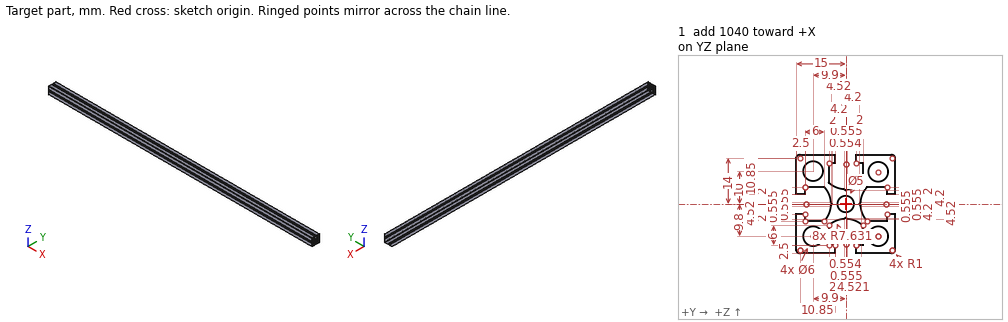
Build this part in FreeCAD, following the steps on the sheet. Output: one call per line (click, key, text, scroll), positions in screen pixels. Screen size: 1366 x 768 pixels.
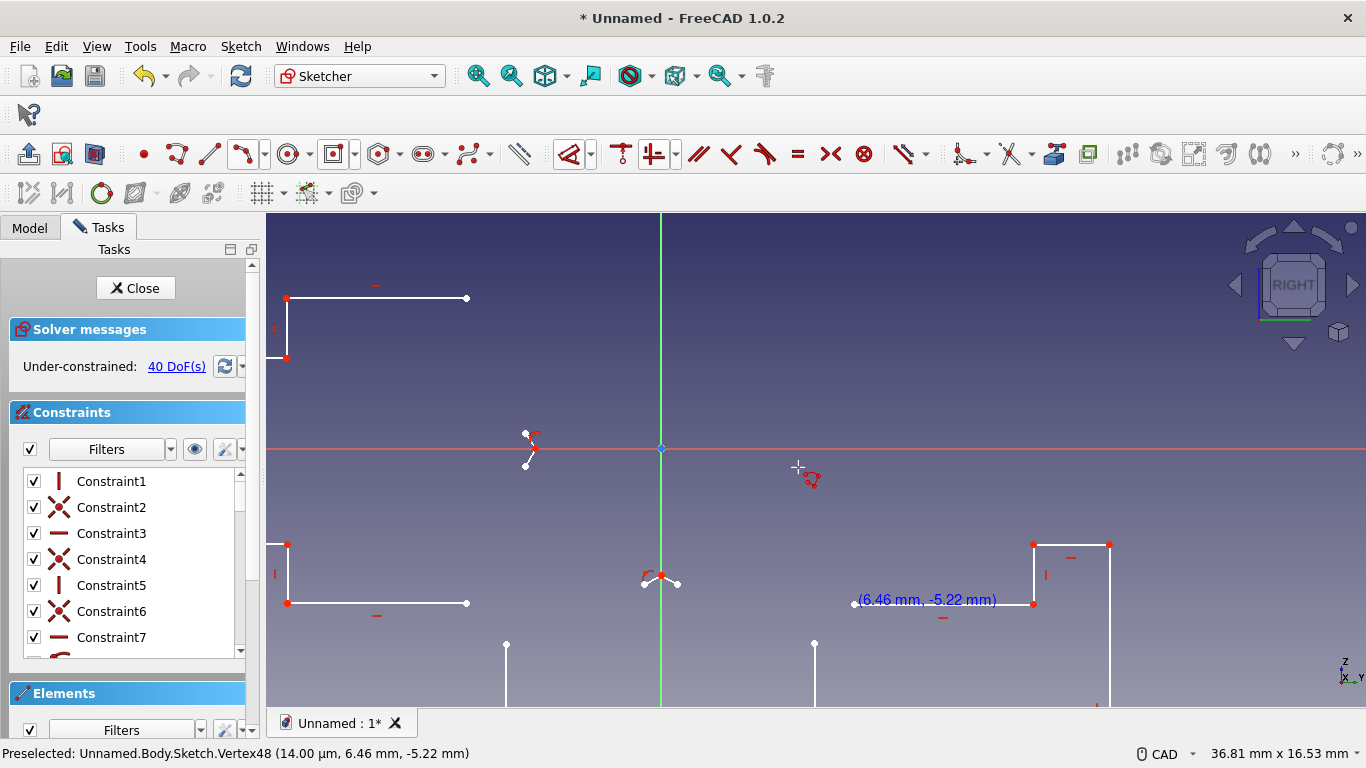
click(796, 465)
click(787, 449)
click(796, 432)
right_click(796, 432)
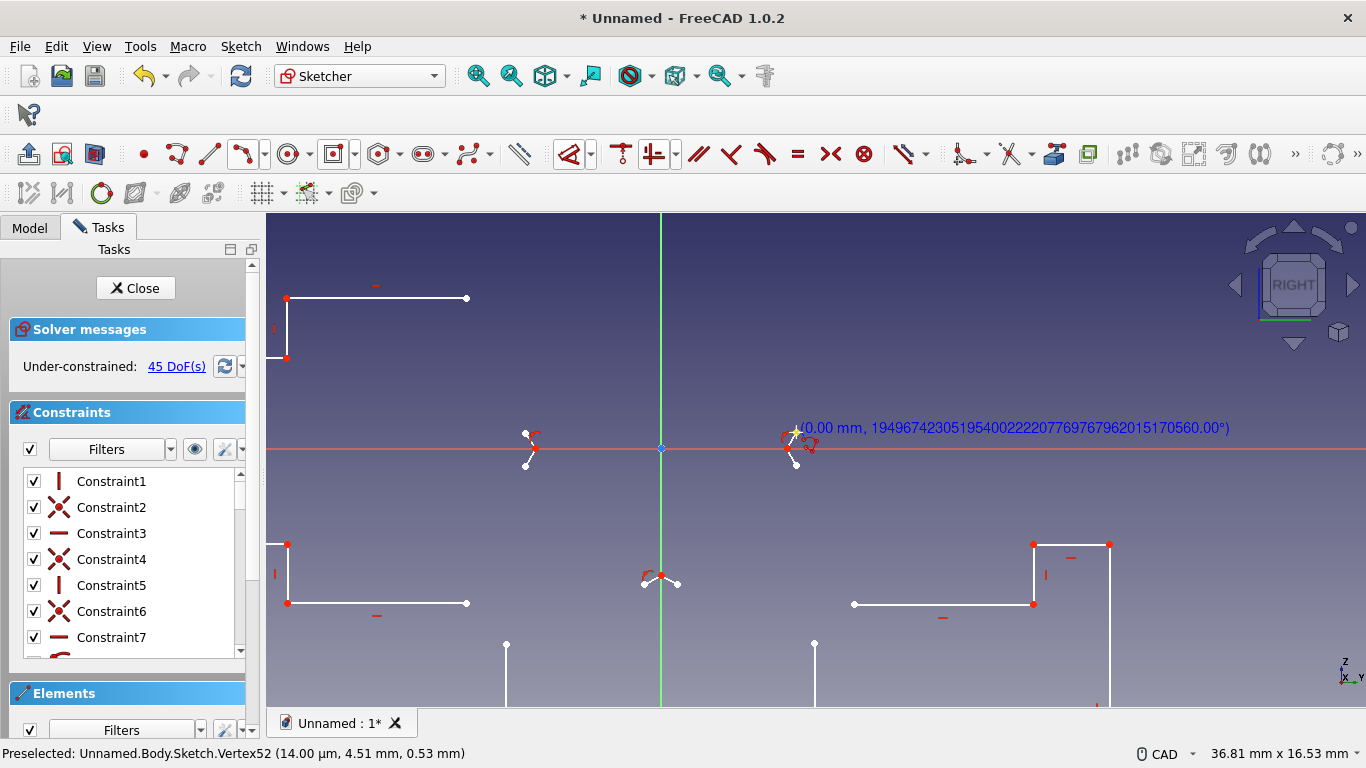
click(855, 295)
click(1035, 295)
click(1035, 355)
click(1109, 355)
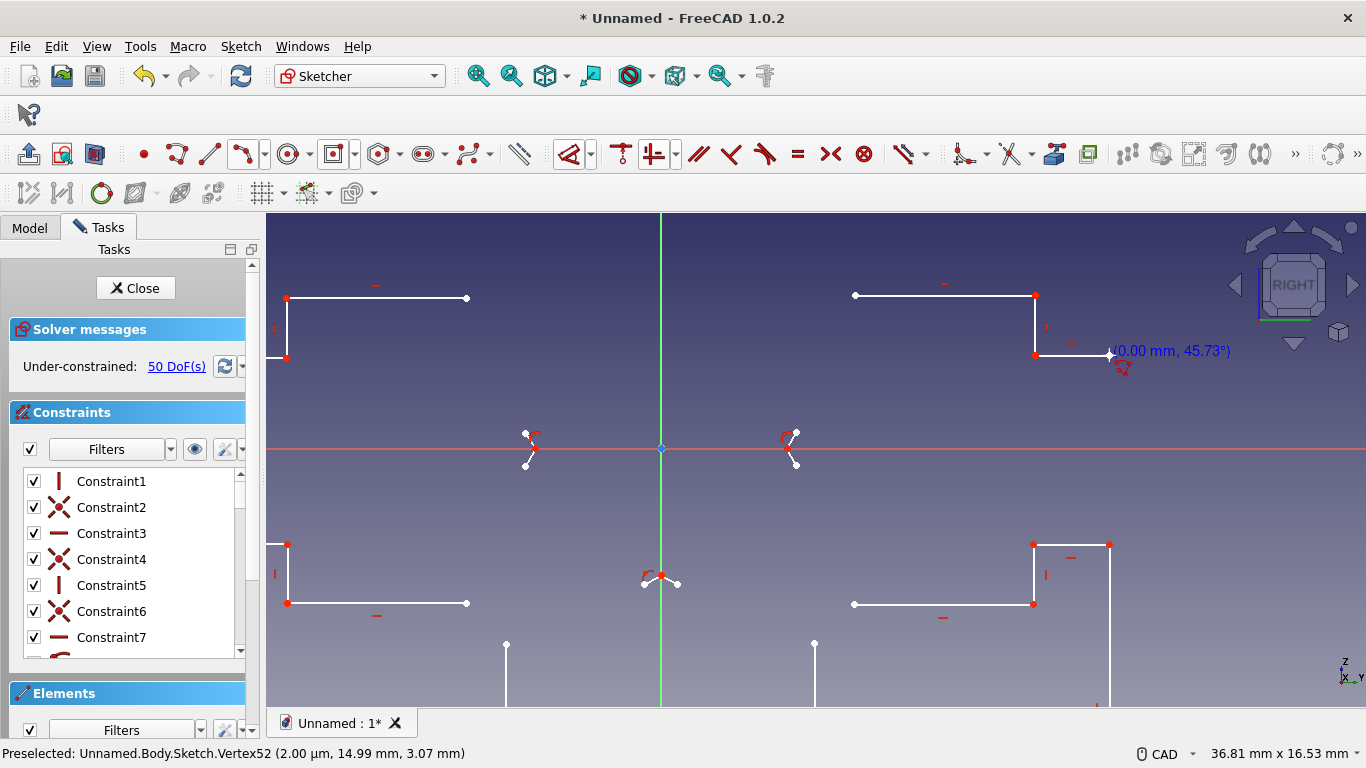
scroll(798, 466, down, 5)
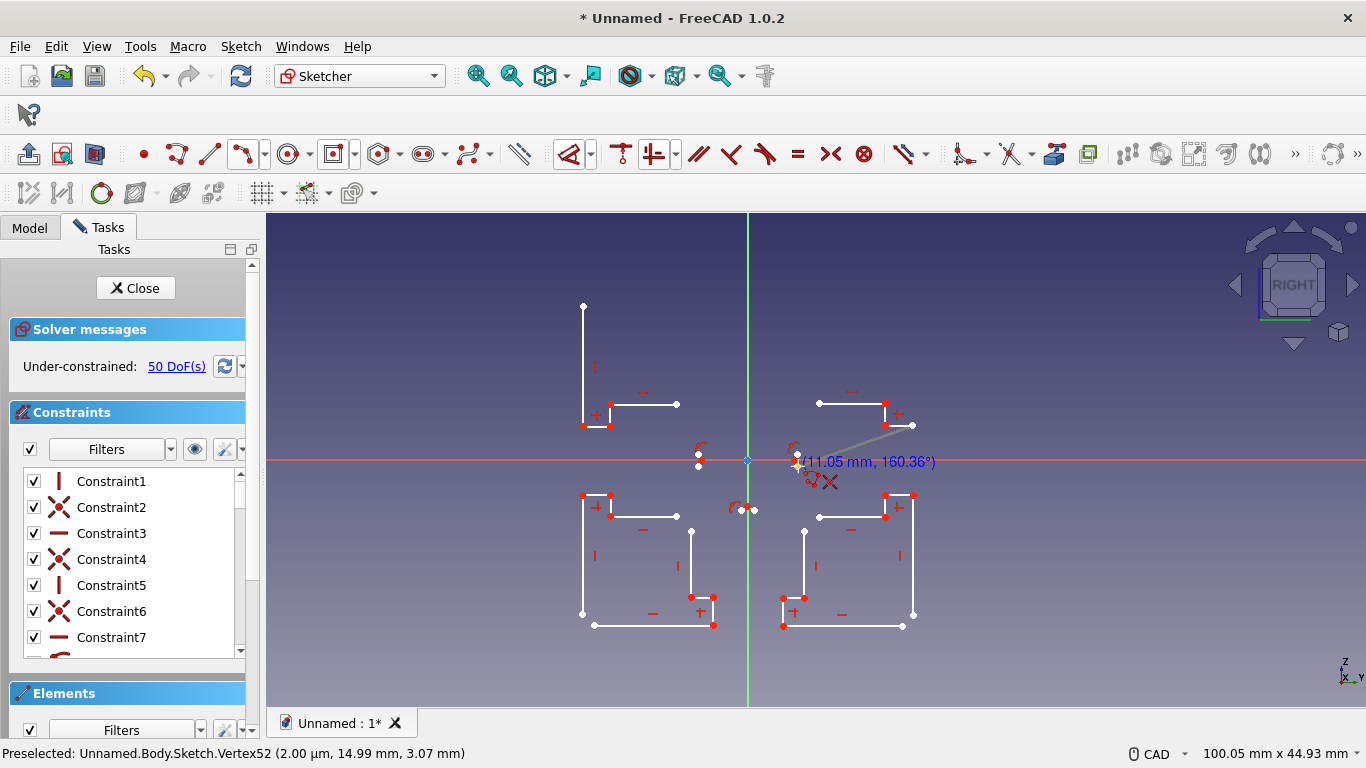
click(913, 306)
right_click(913, 306)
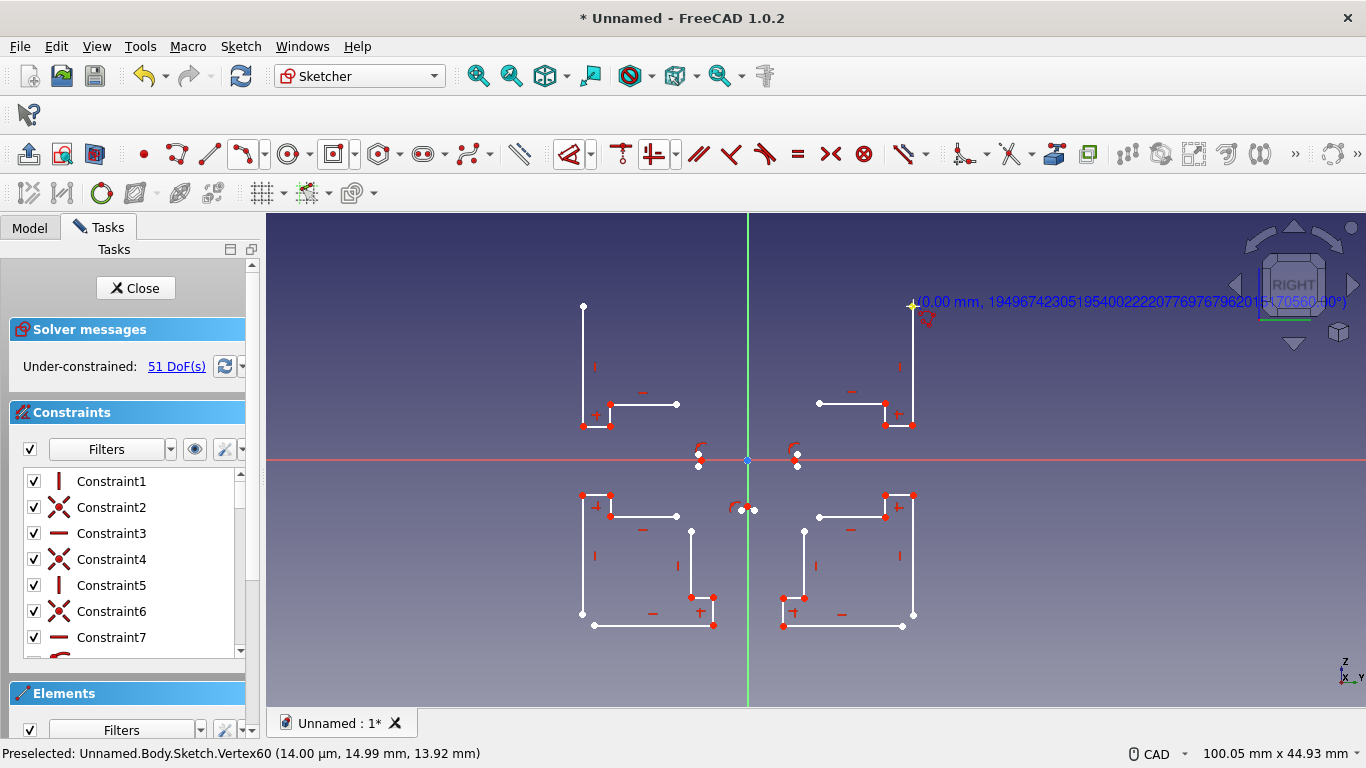
click(902, 295)
click(783, 295)
click(783, 323)
click(805, 323)
click(805, 389)
right_click(805, 389)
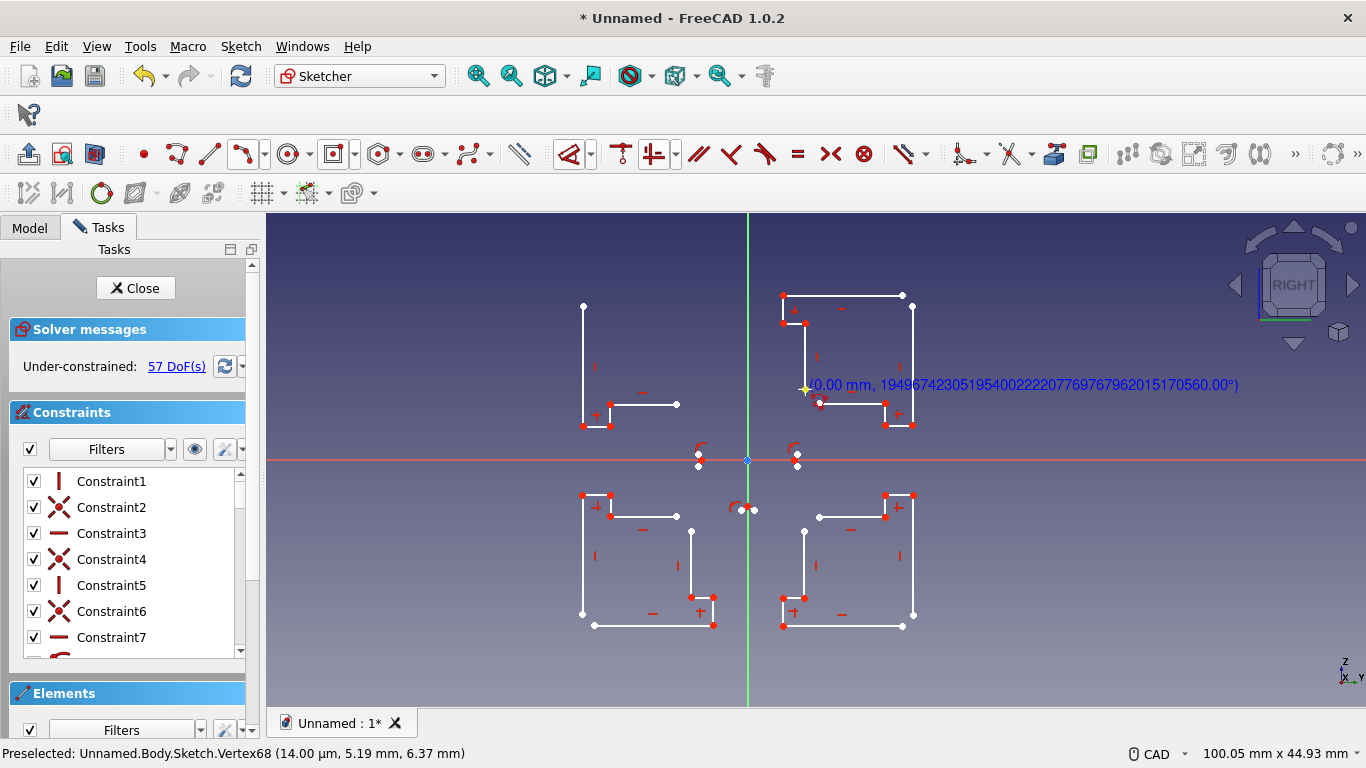
scroll(754, 410, up, 5)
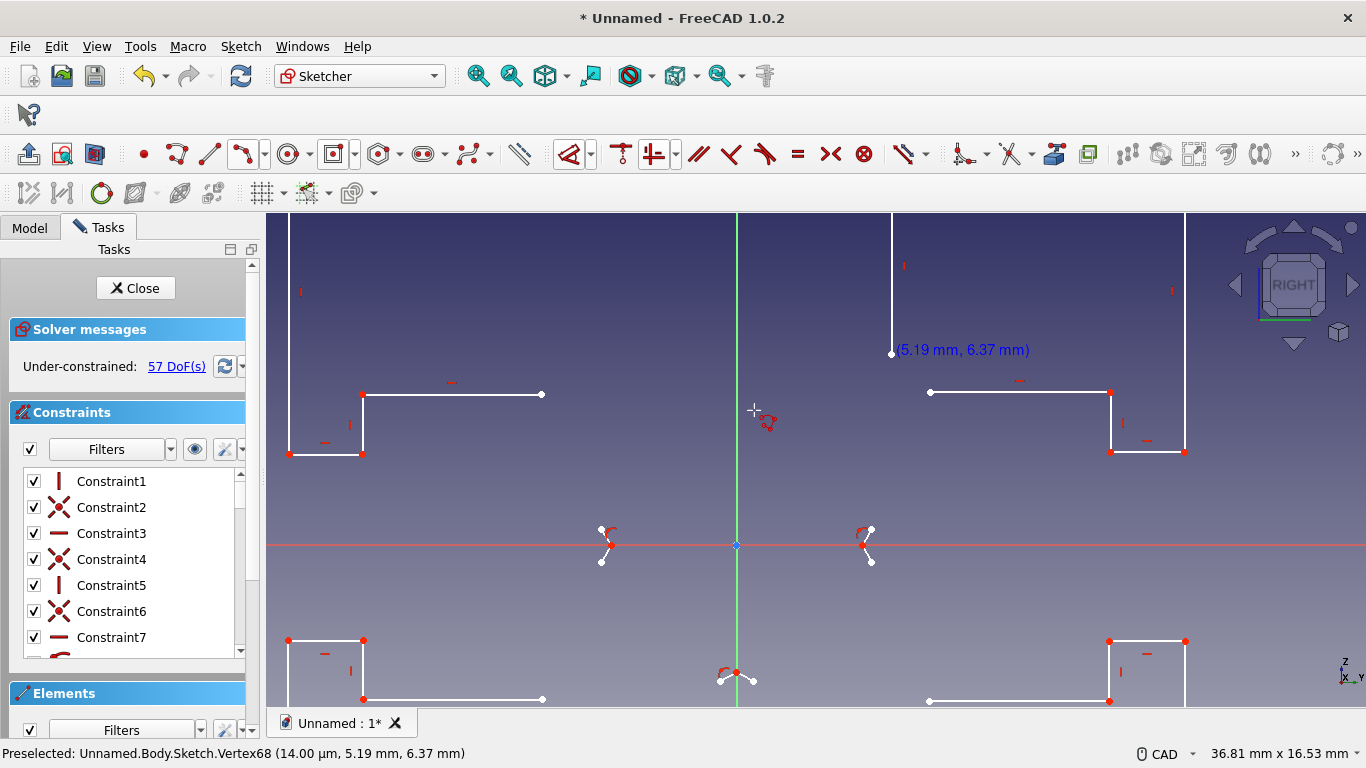
click(753, 410)
click(737, 420)
click(720, 410)
right_click(720, 410)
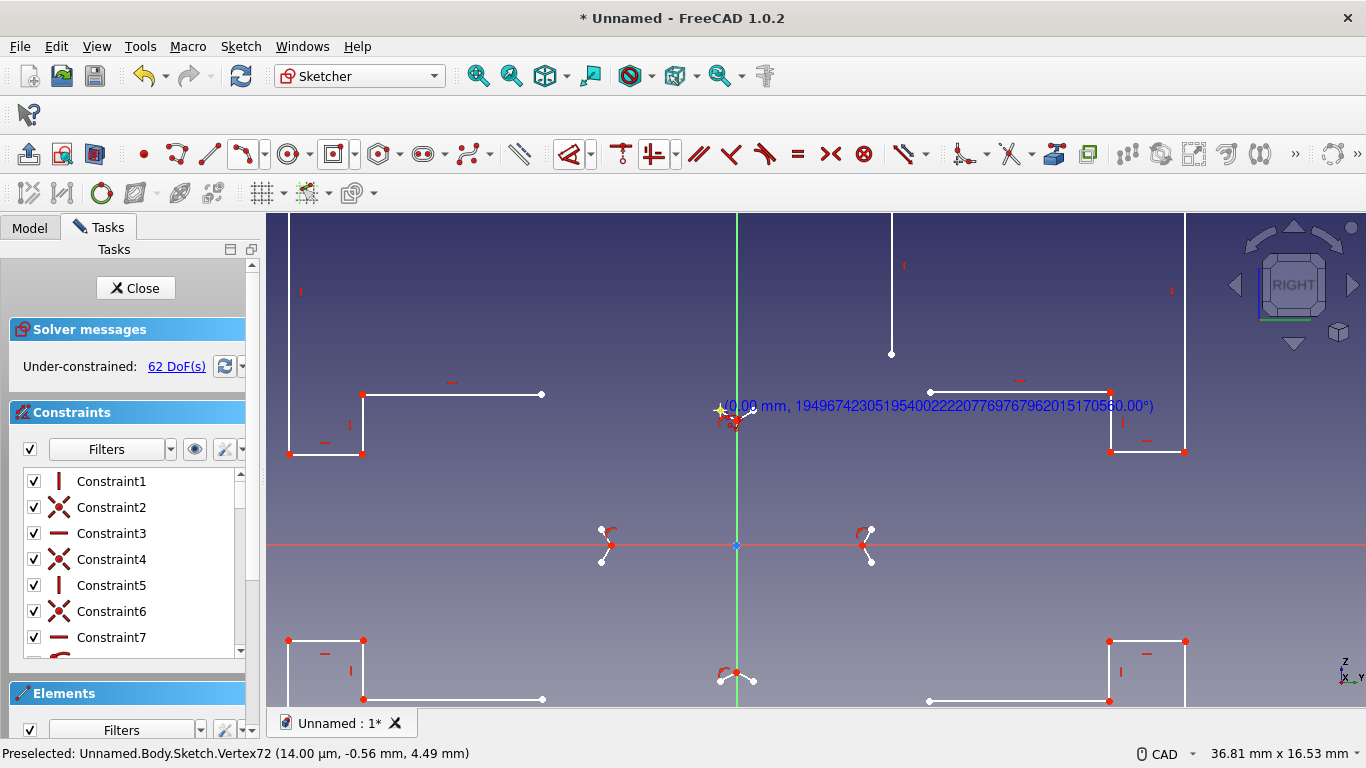
click(583, 351)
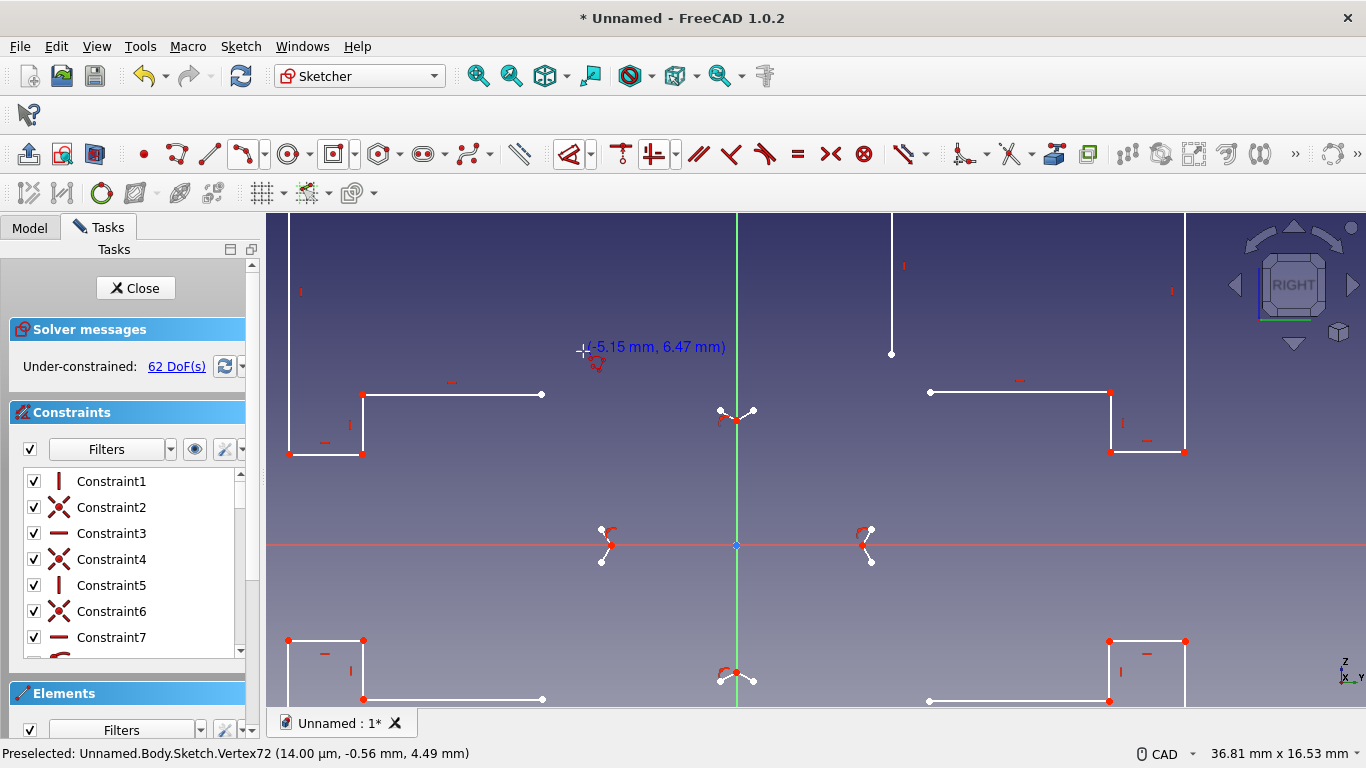
scroll(754, 410, down, 5)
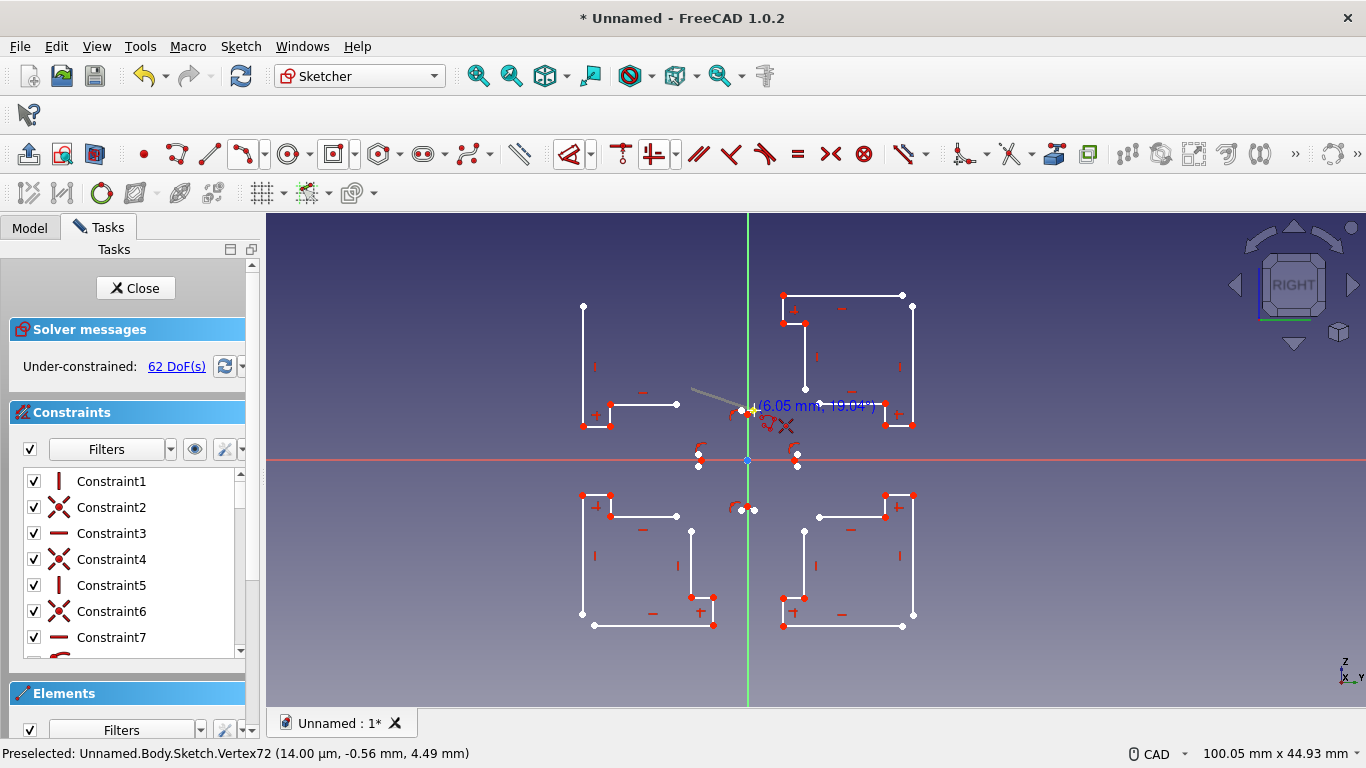
click(691, 323)
click(713, 323)
click(713, 295)
click(594, 295)
right_click(594, 295)